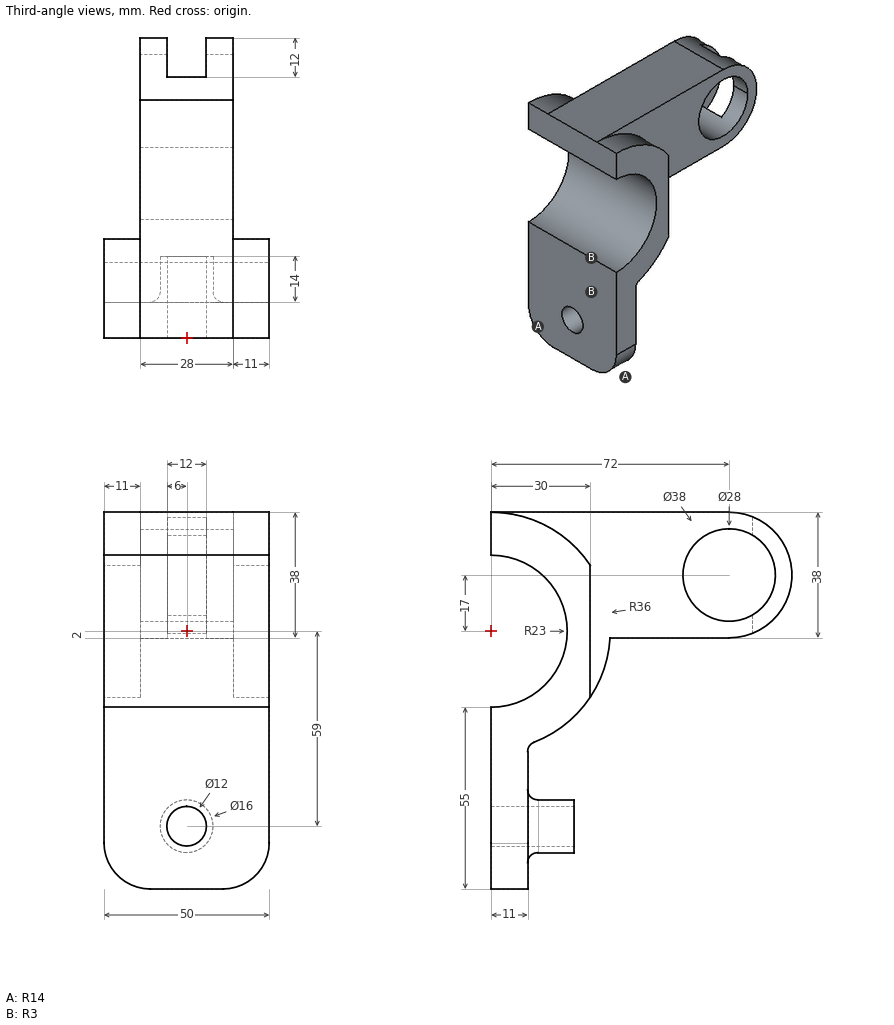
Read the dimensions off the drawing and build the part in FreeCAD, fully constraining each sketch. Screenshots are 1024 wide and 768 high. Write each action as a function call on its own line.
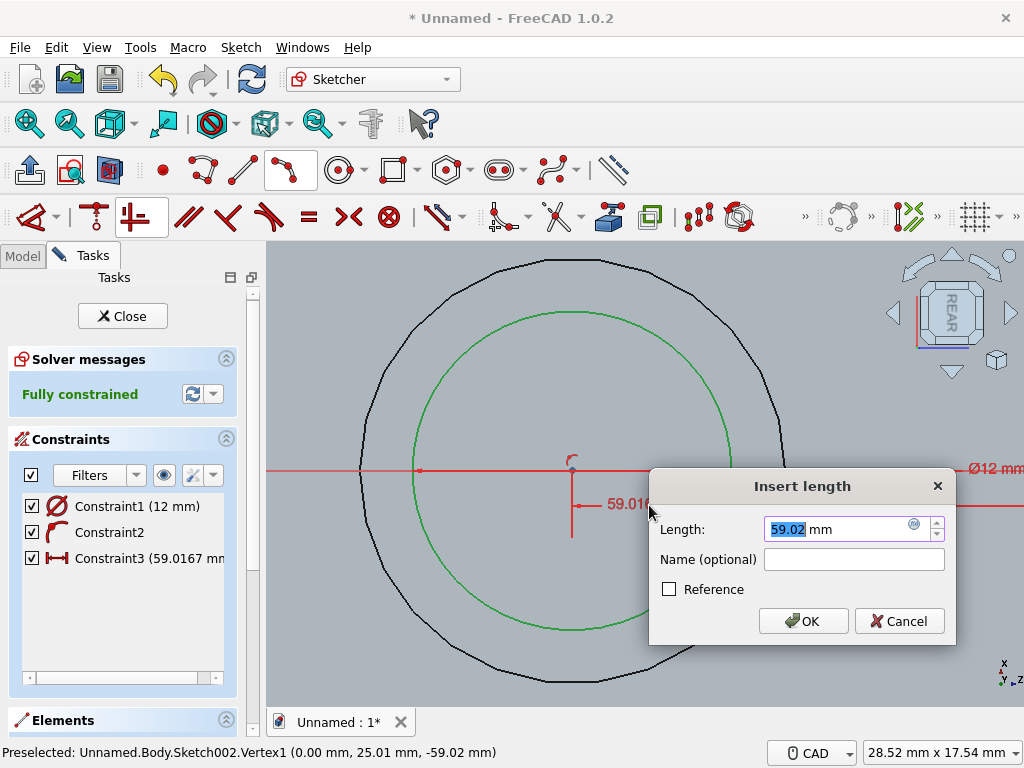
text(59)
key(Return)
key(Escape)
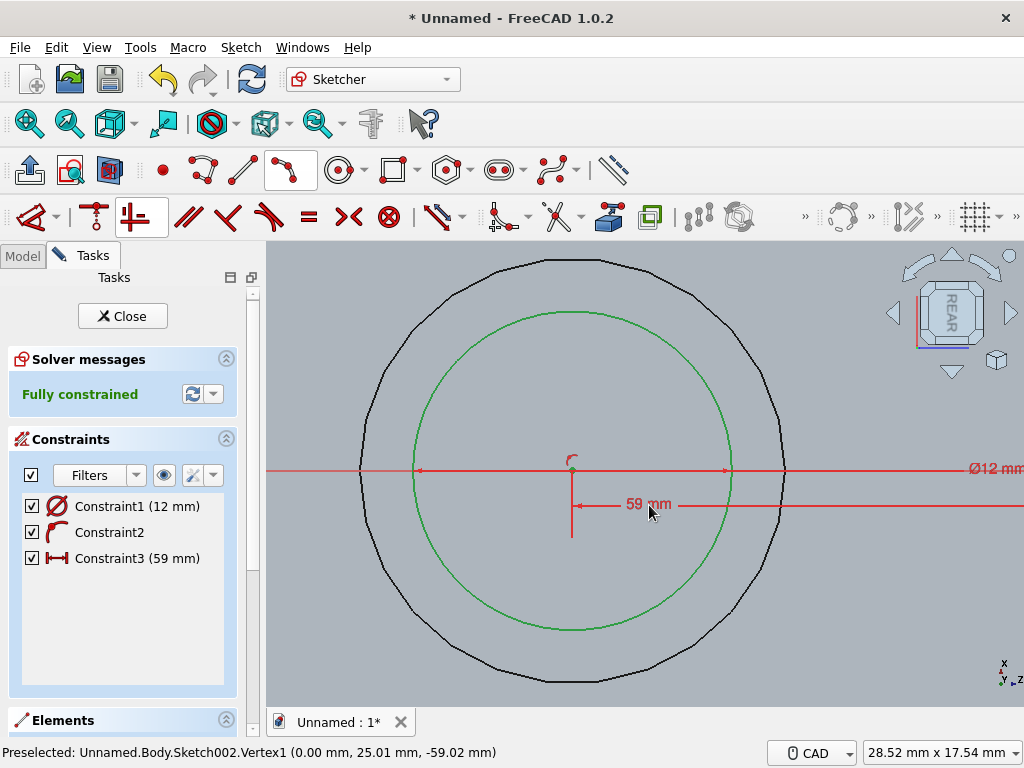
click(123, 316)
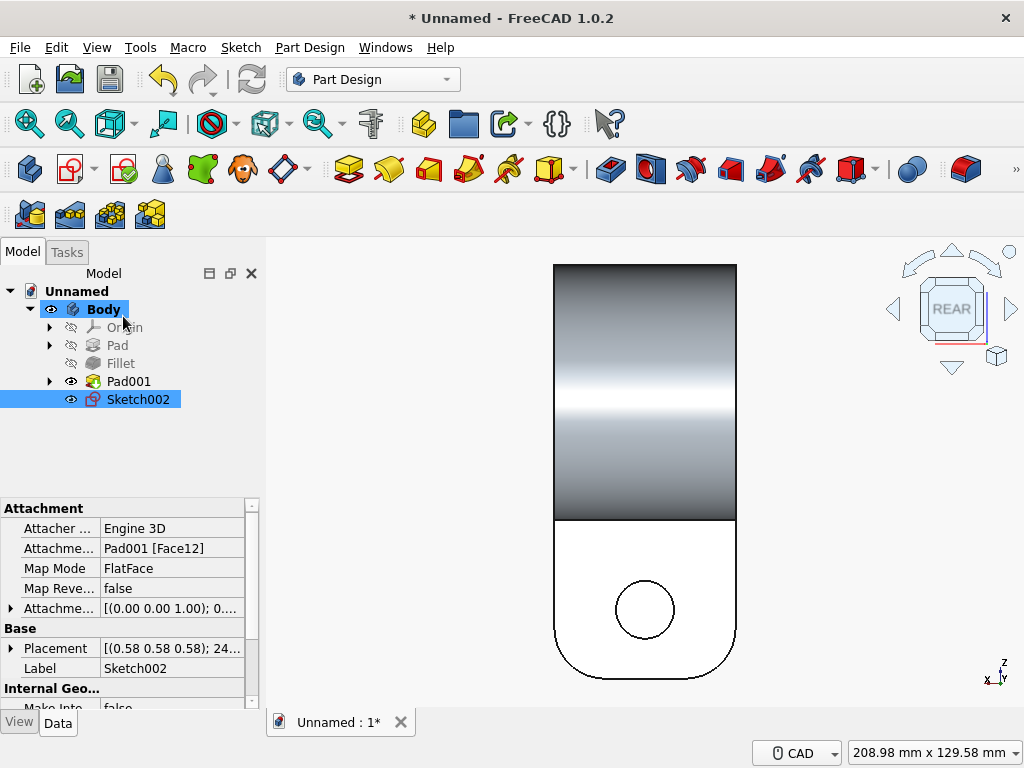
click(612, 170)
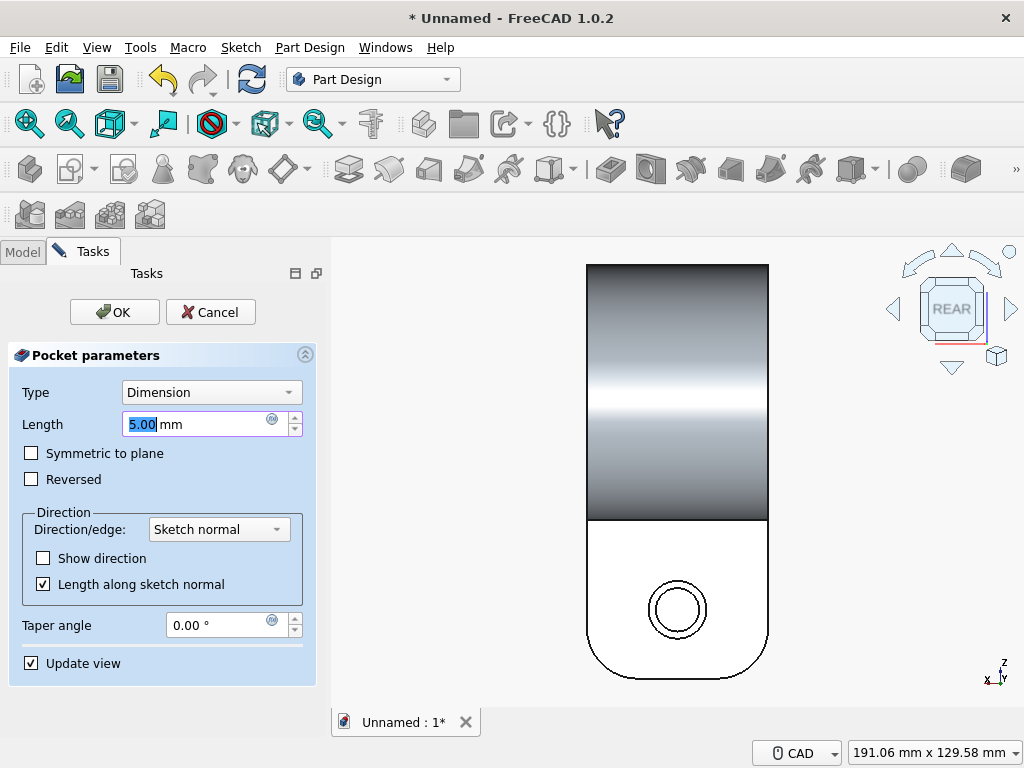
click(212, 392)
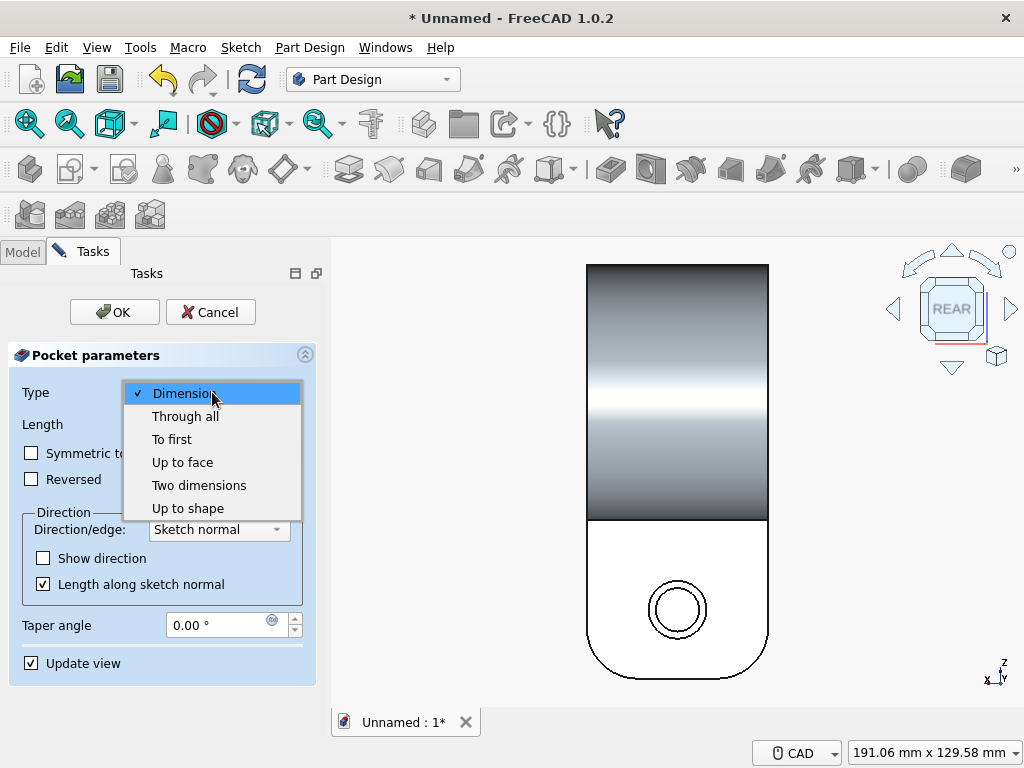
click(212, 416)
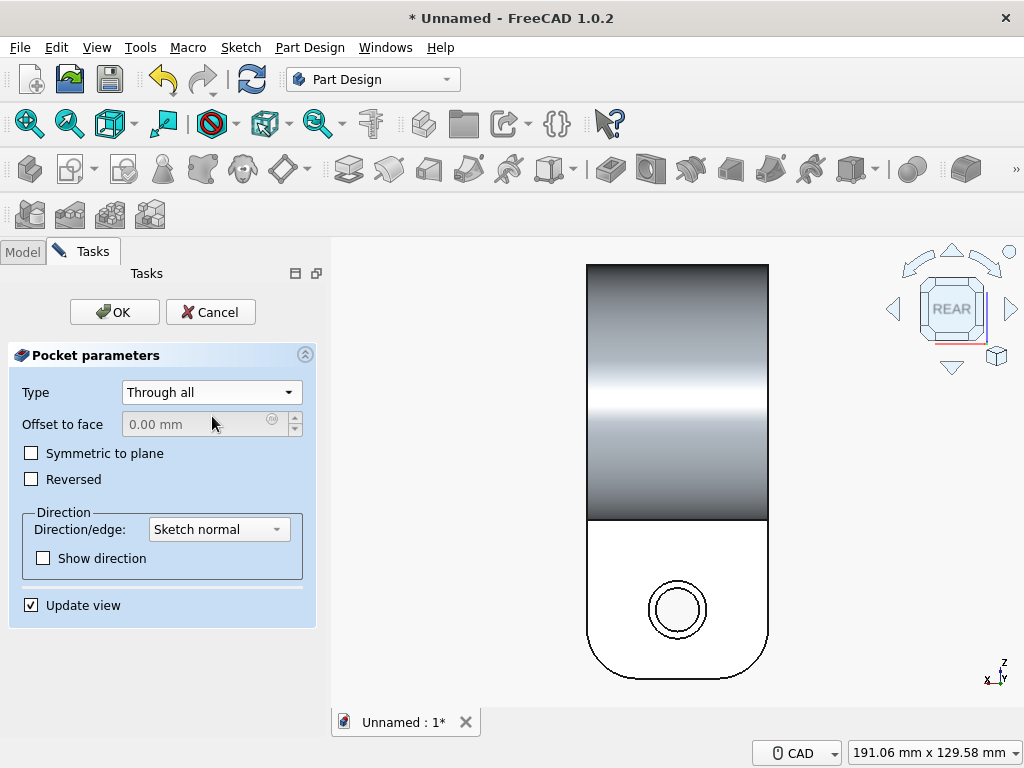
click(115, 312)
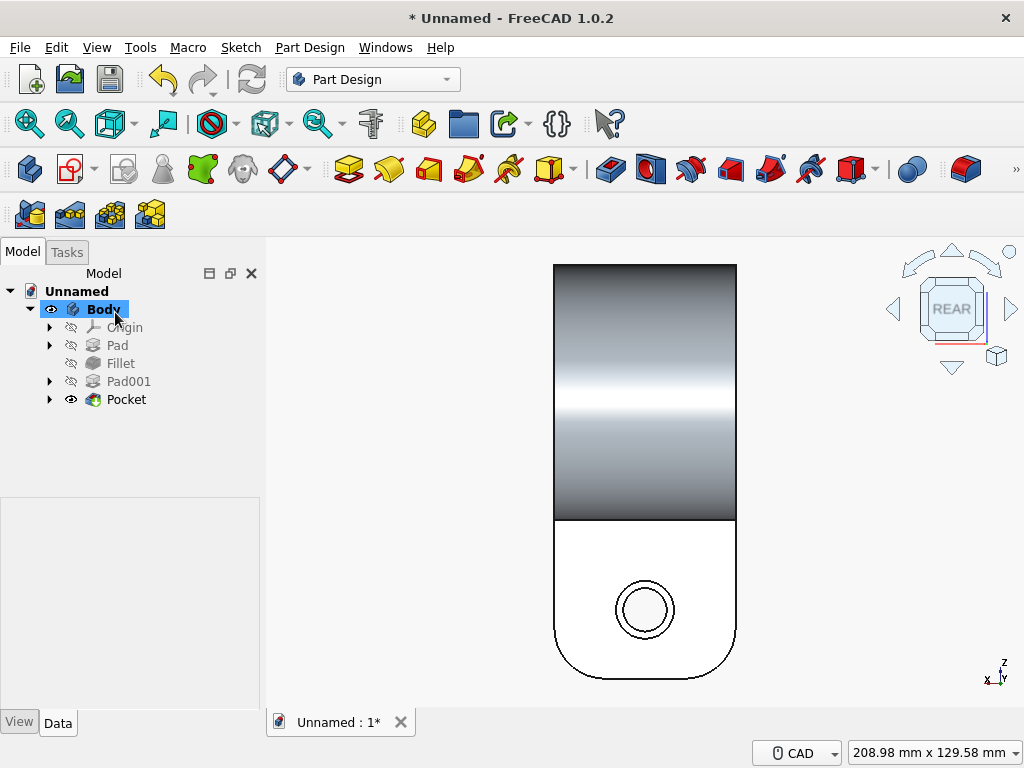
key(0)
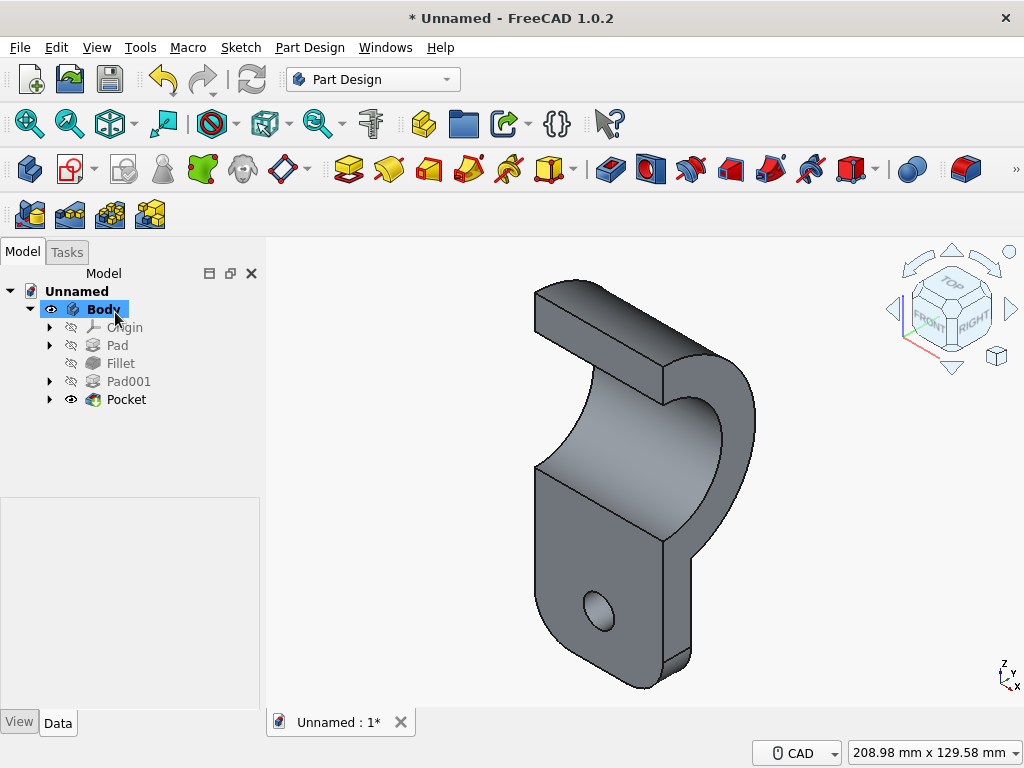
key(2)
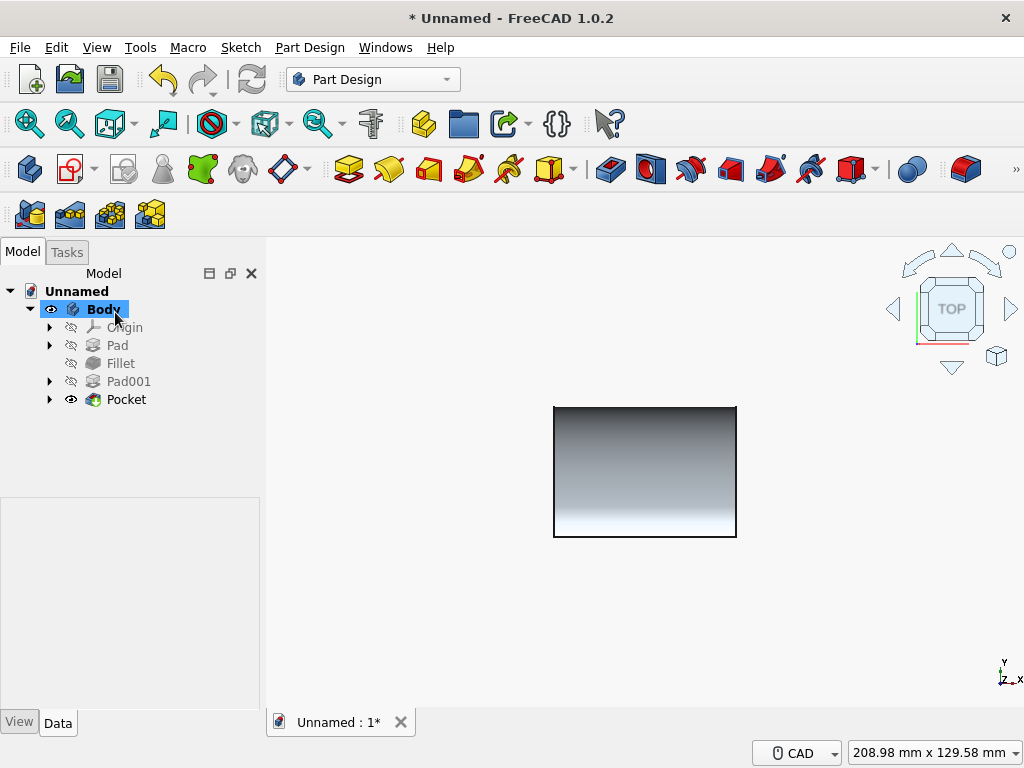
click(30, 124)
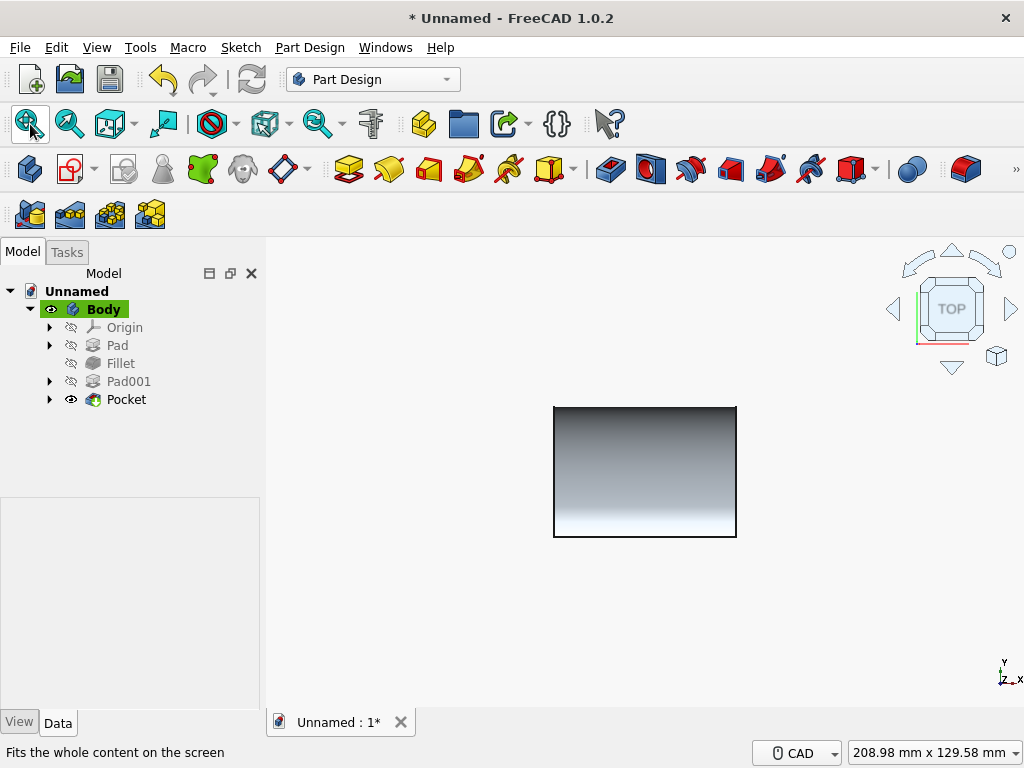
key(1)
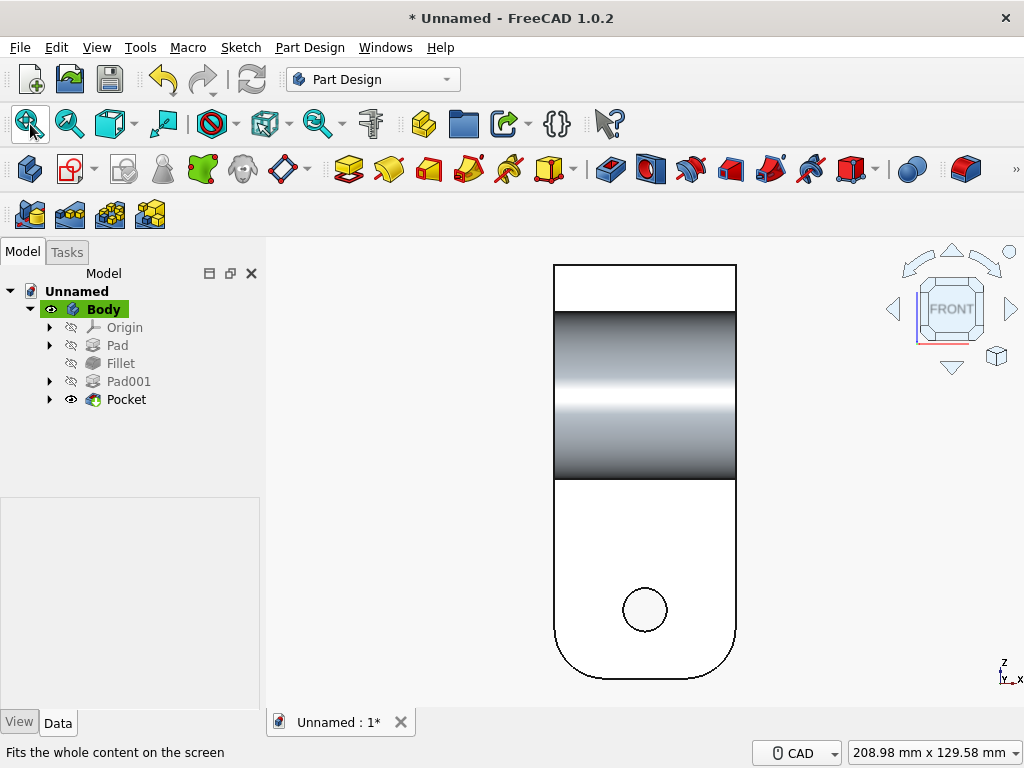
key(3)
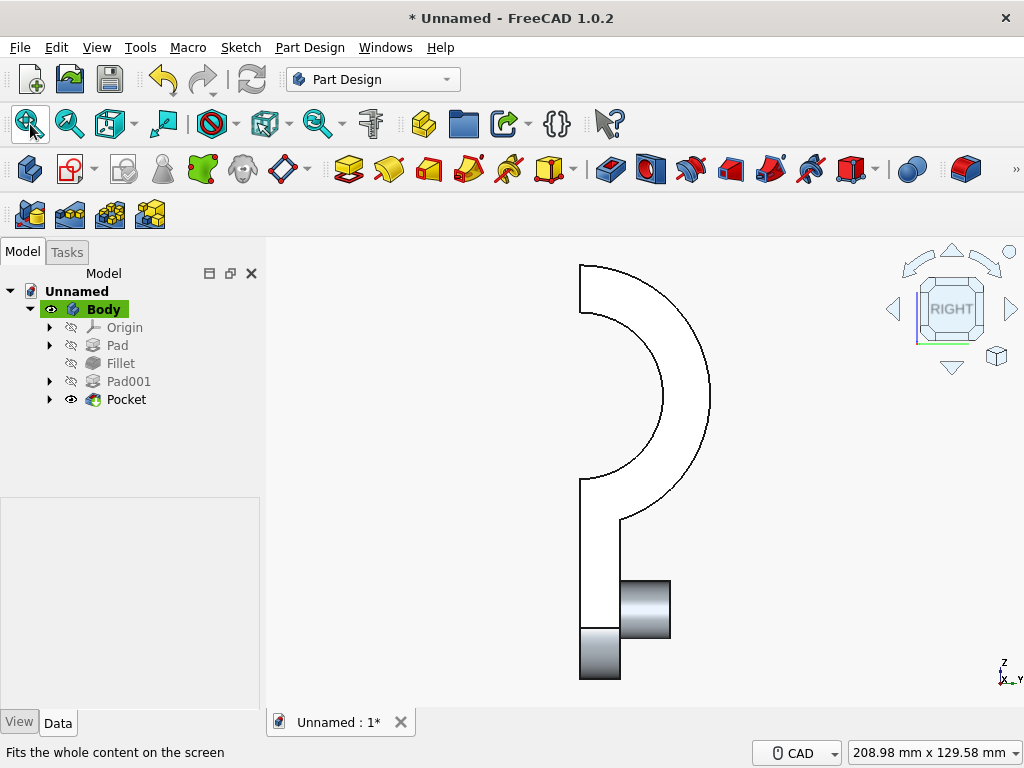
key(5)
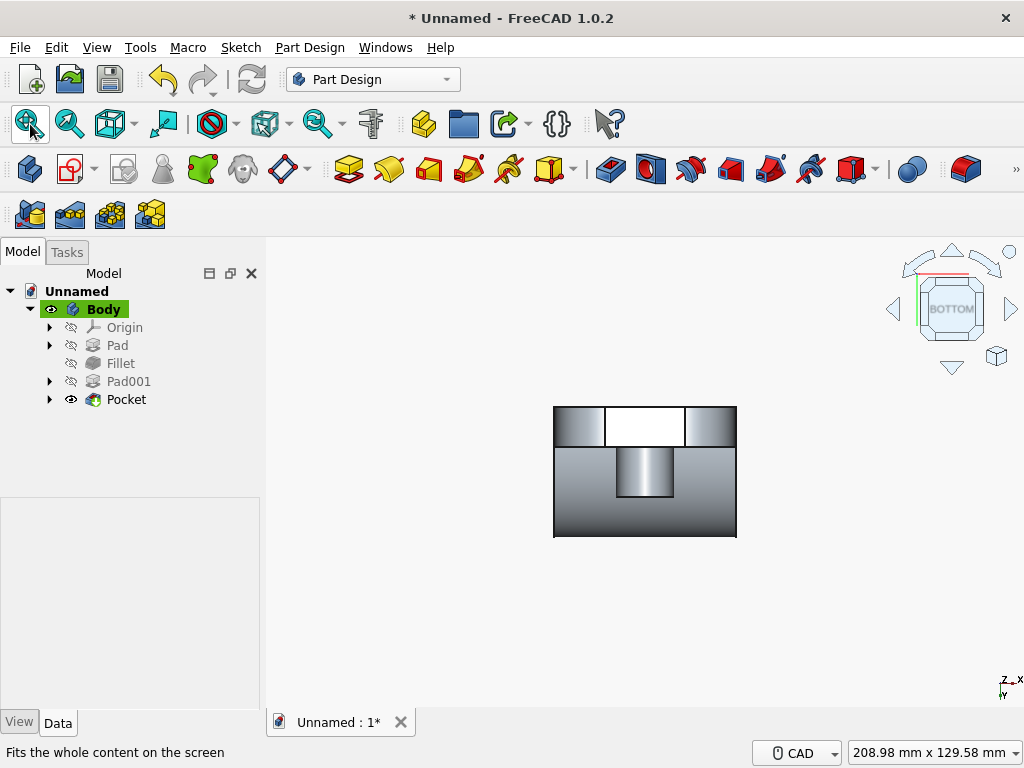
click(30, 124)